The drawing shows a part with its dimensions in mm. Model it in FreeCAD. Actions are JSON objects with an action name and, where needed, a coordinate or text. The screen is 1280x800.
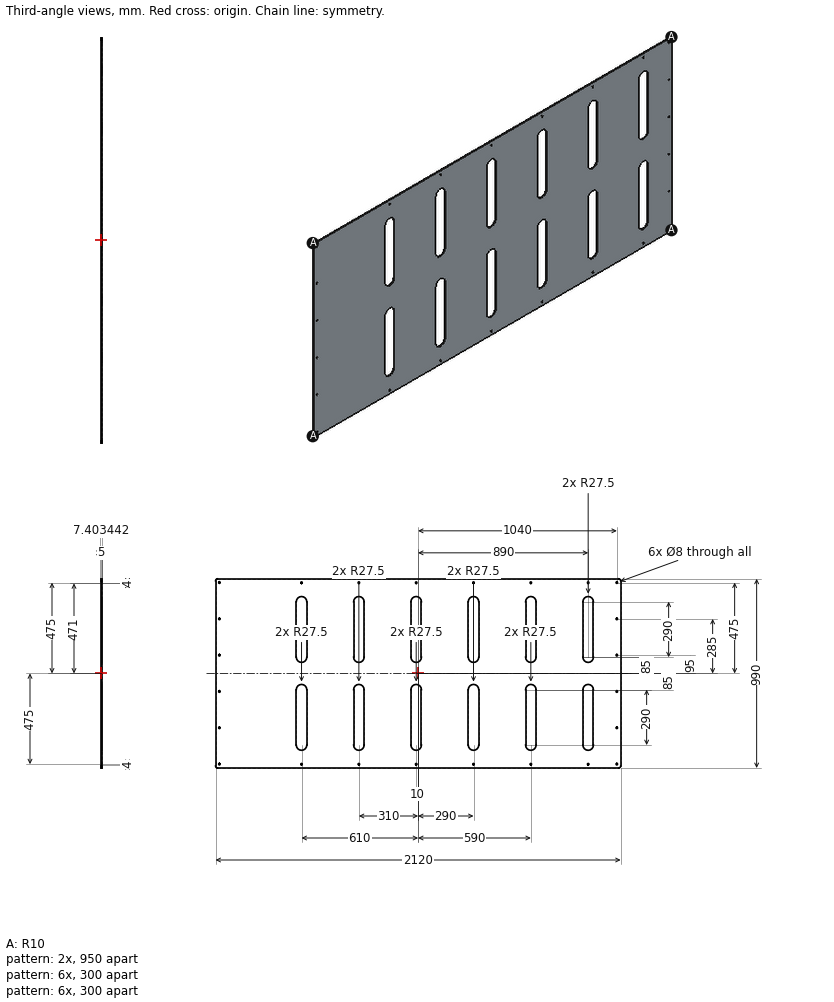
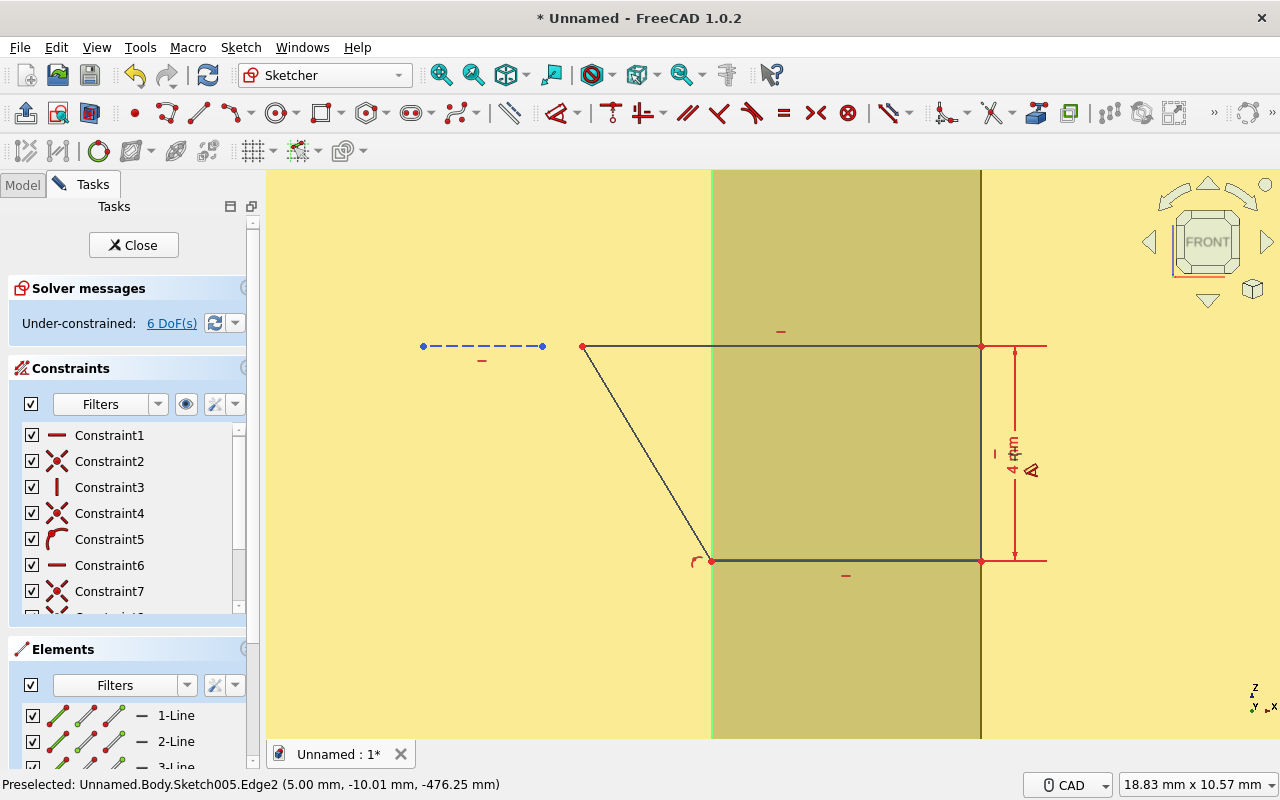
{"action": "left_click", "coordinate": [900, 561]}
{"action": "left_click", "coordinate": [846, 595]}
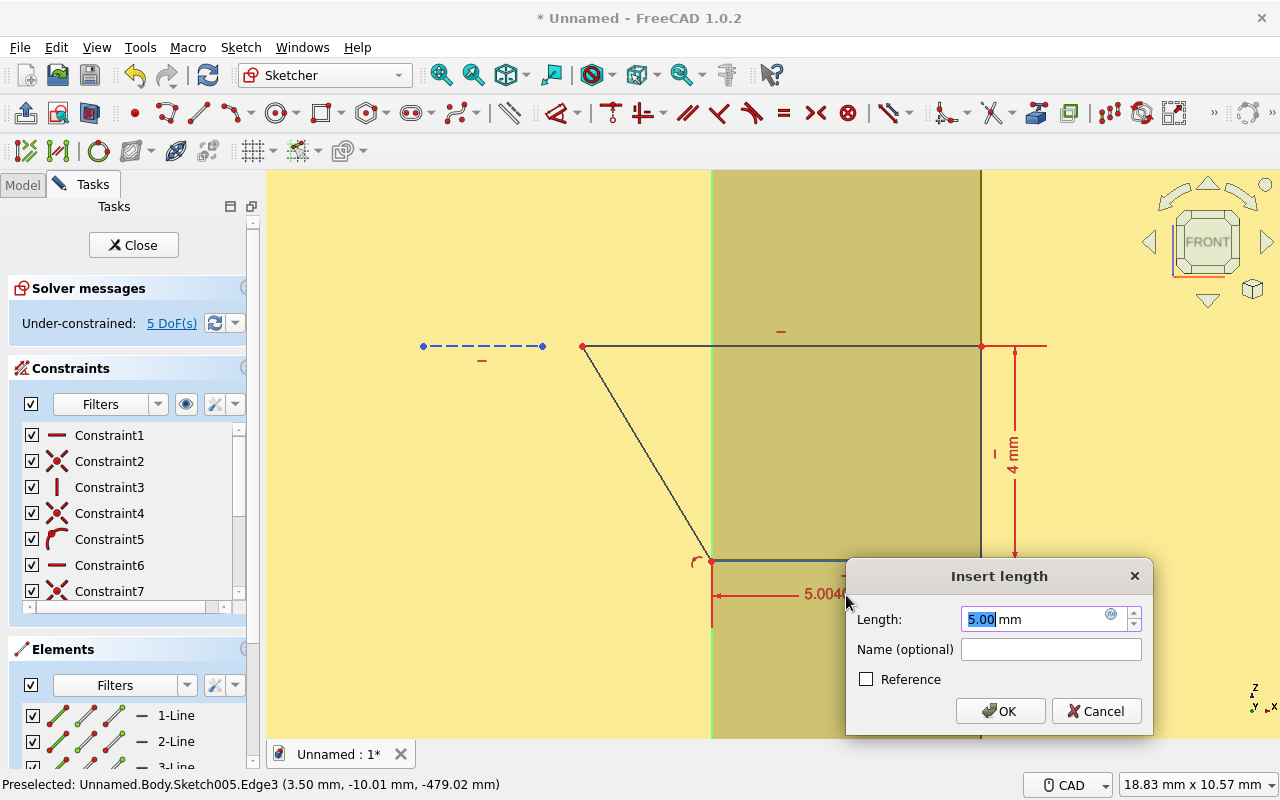
{"action": "type", "text": "5"}
{"action": "key", "text": "Return"}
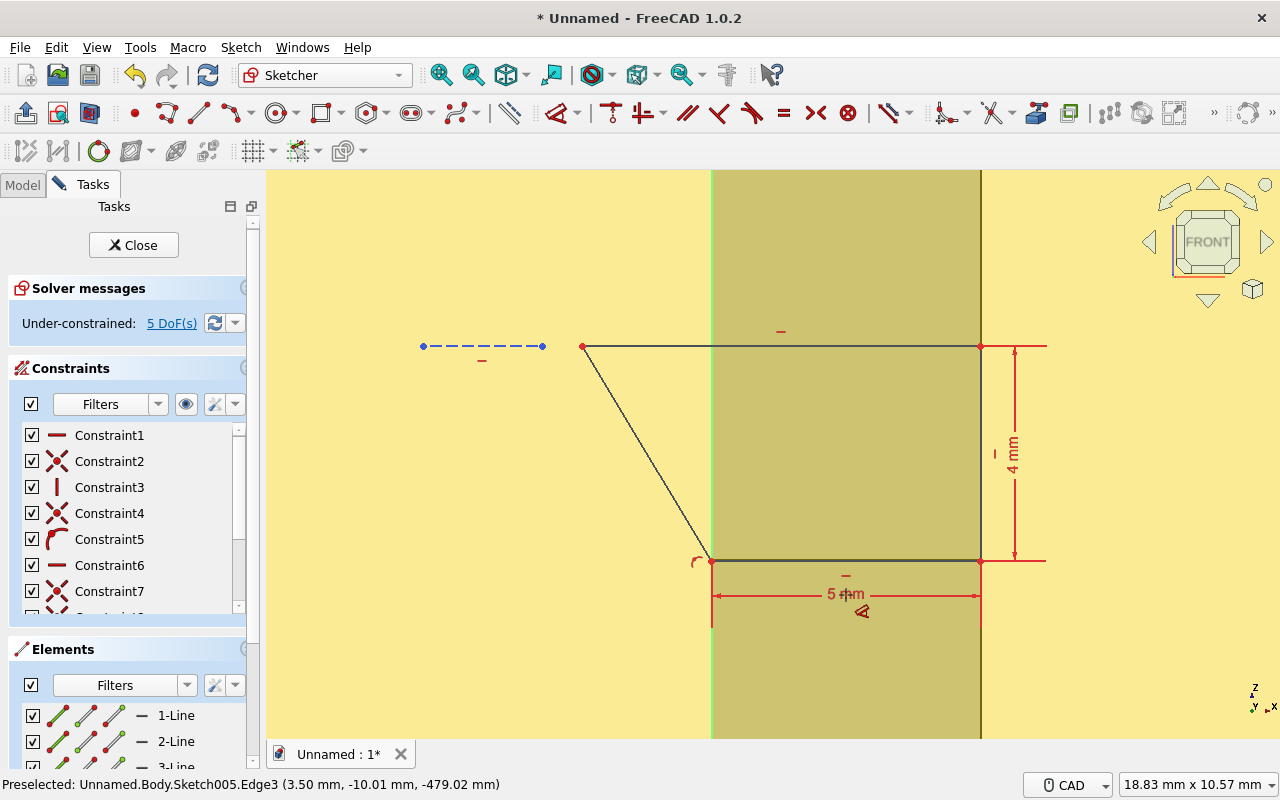
{"action": "left_click", "coordinate": [582, 346]}
{"action": "left_click", "coordinate": [548, 272]}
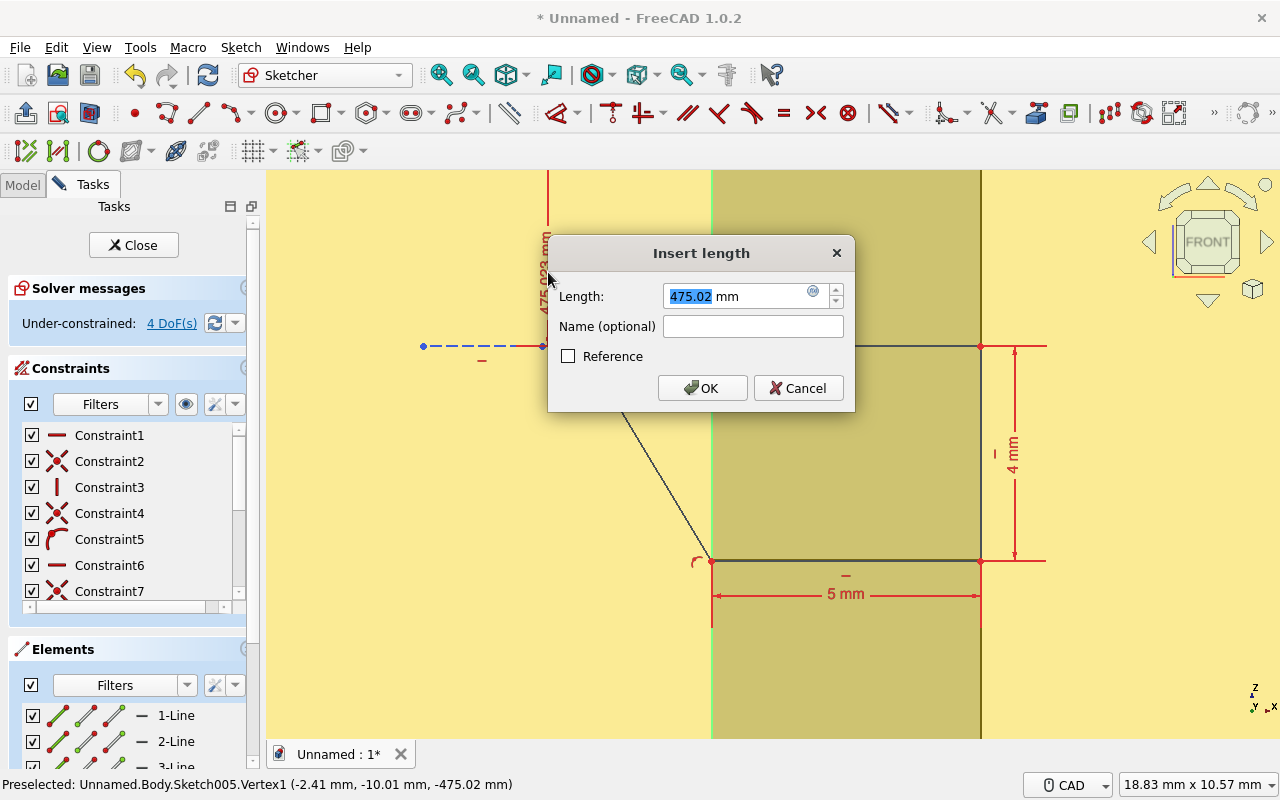
{"action": "type", "text": "475"}
{"action": "key", "text": "Return"}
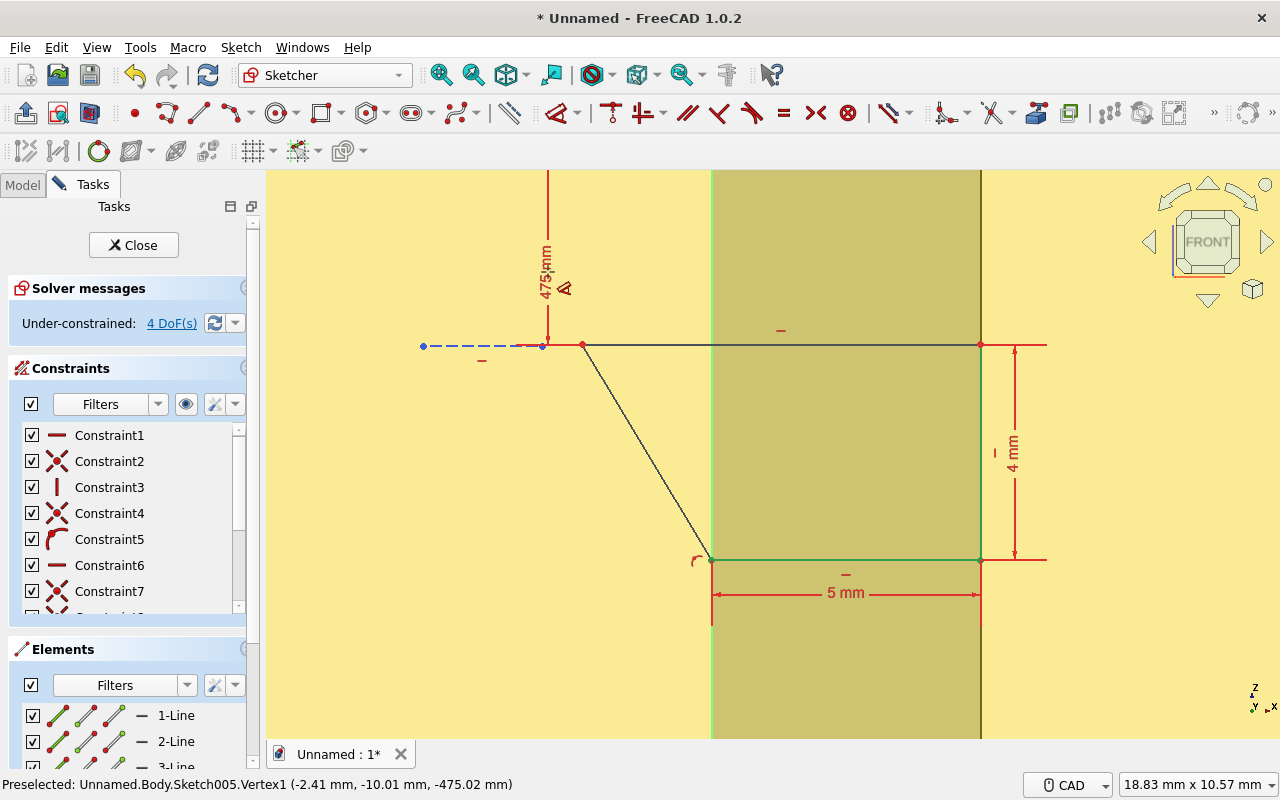
{"action": "left_click", "coordinate": [542, 346]}
{"action": "left_click", "coordinate": [508, 238]}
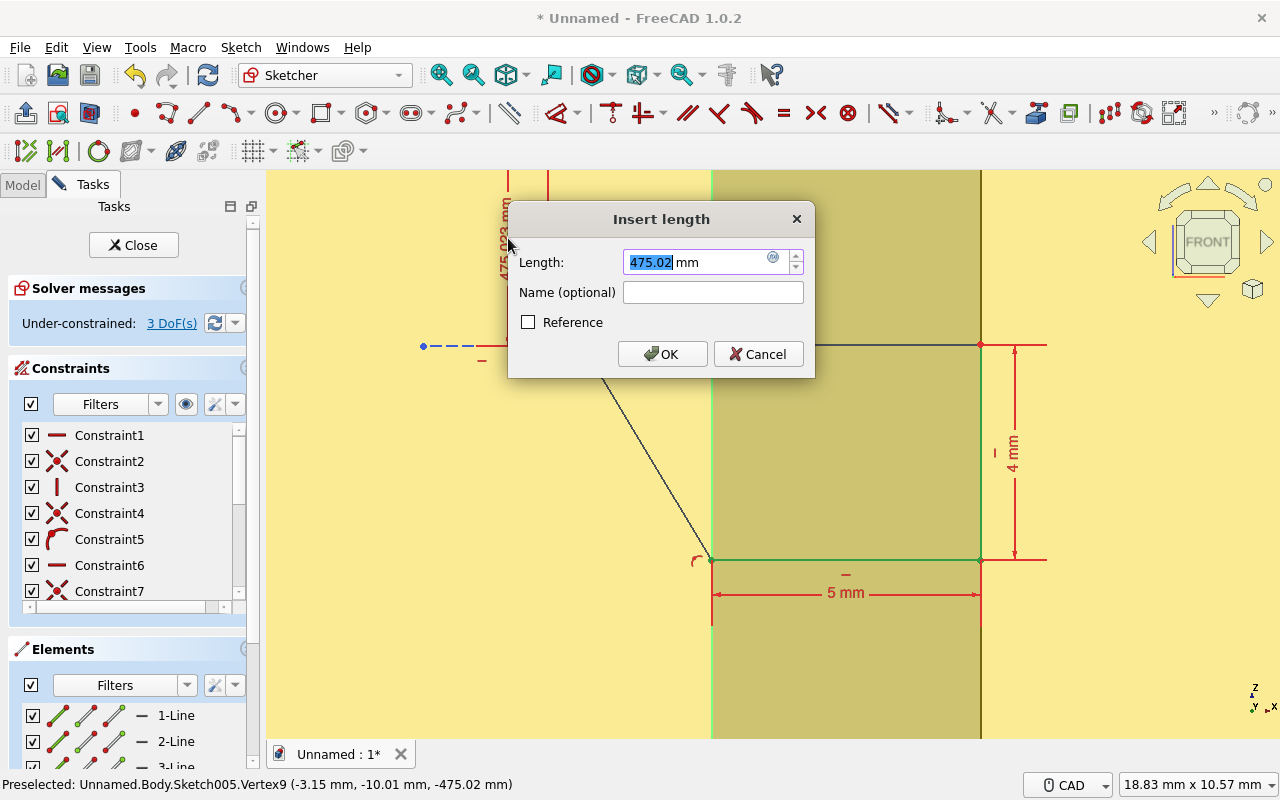
{"action": "type", "text": "475"}
{"action": "key", "text": "Return"}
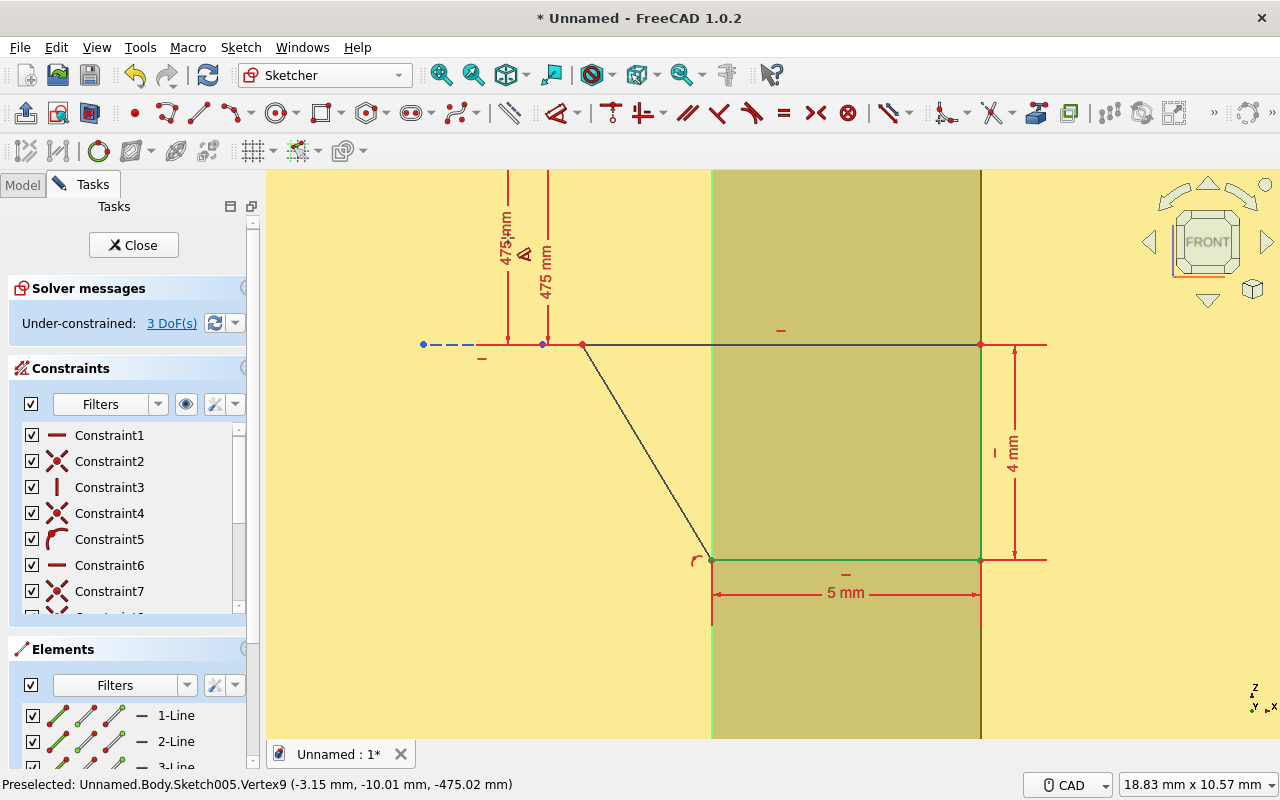
{"action": "scroll", "coordinate": [702, 345], "scroll_direction": "up", "scroll_amount": 2}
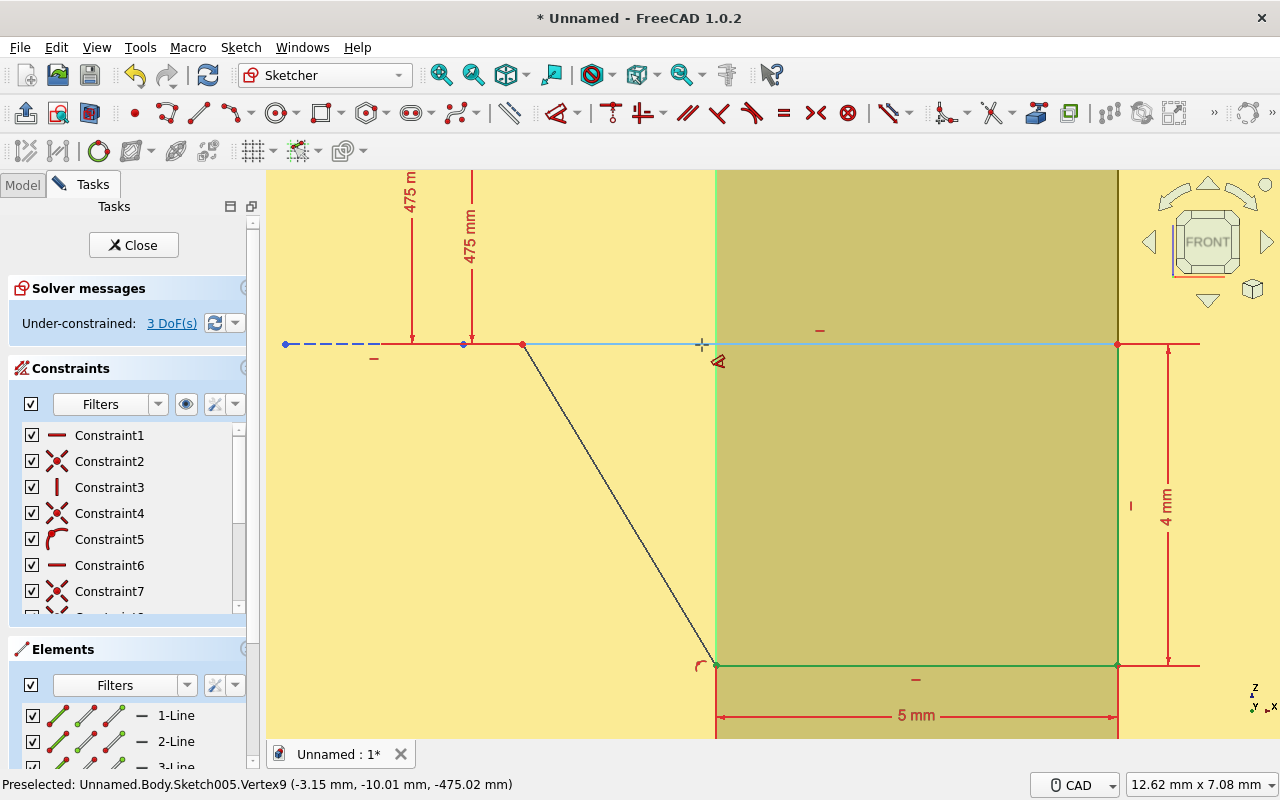
{"action": "left_click", "coordinate": [701, 344]}
{"action": "left_click", "coordinate": [819, 310]}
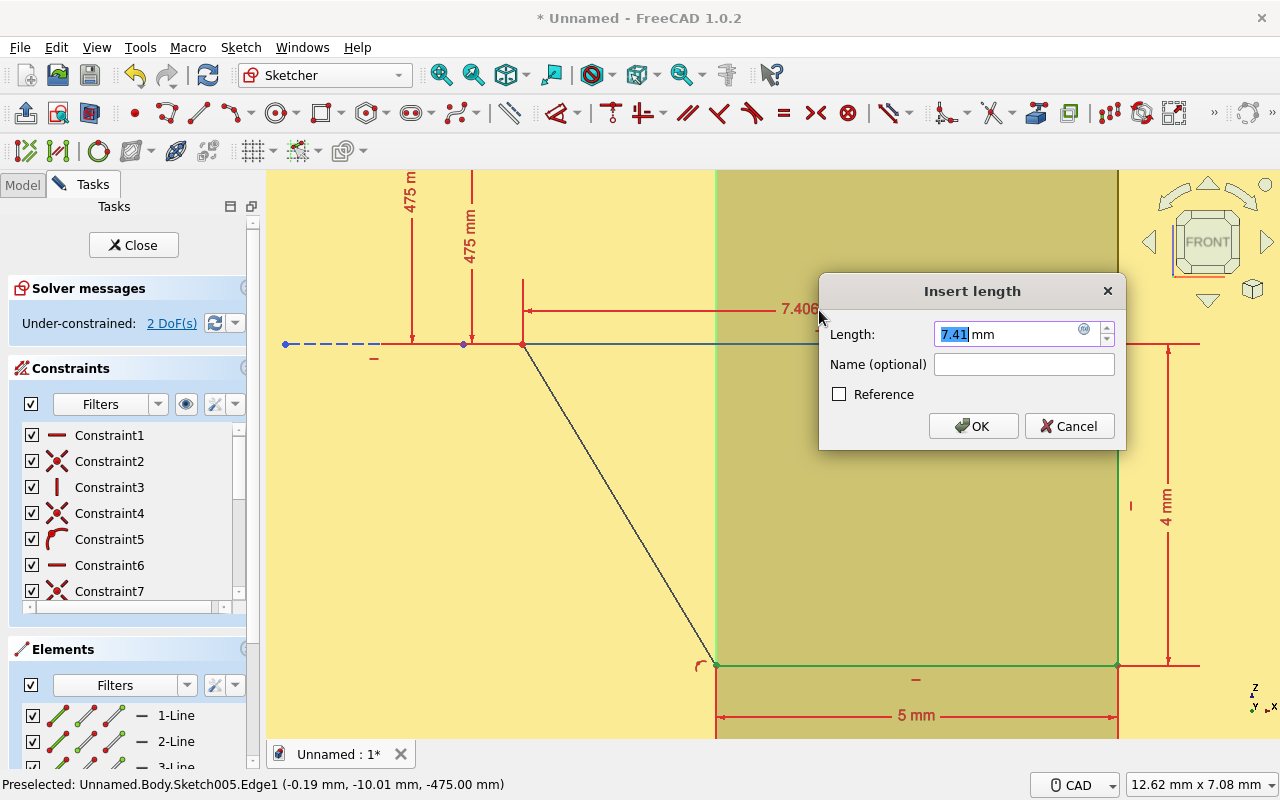
{"action": "type", "text": "7.403442"}
{"action": "key", "text": "Return"}
{"action": "key", "text": "Escape"}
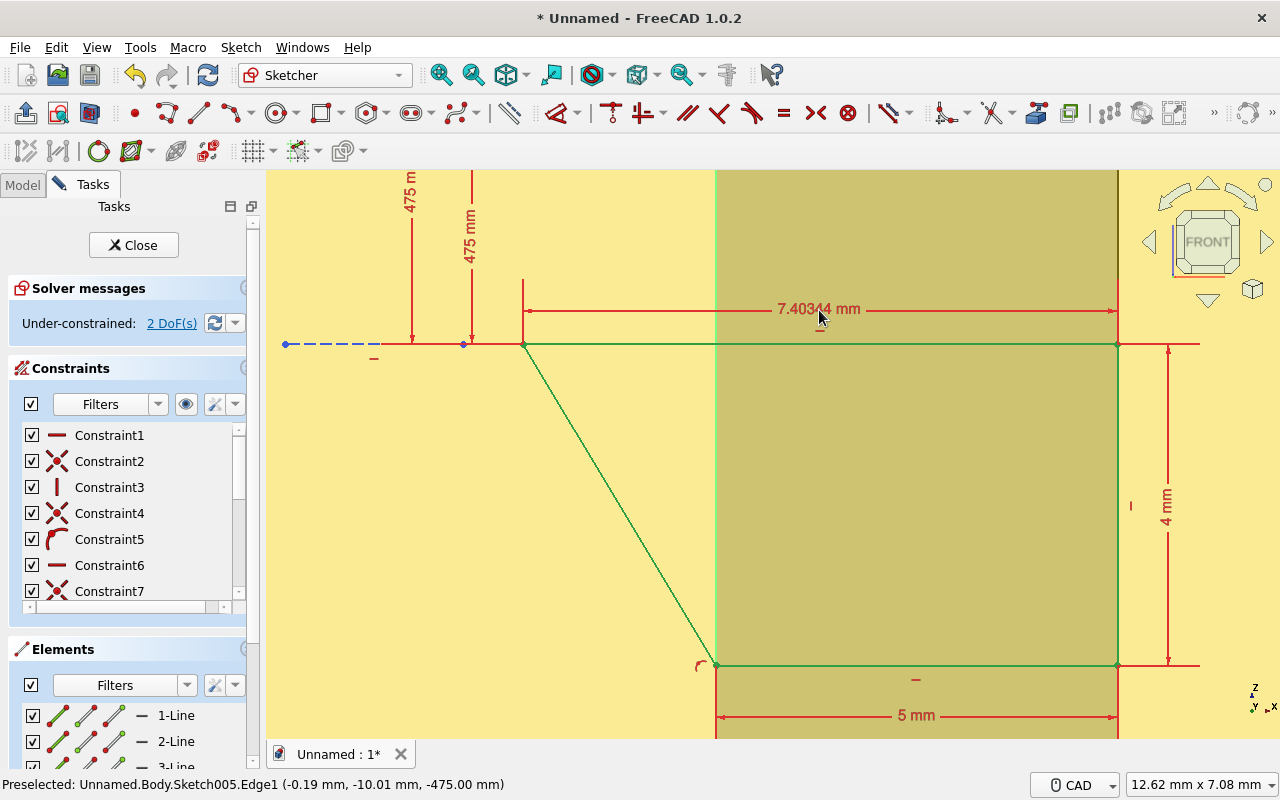
{"action": "left_click", "coordinate": [134, 245]}